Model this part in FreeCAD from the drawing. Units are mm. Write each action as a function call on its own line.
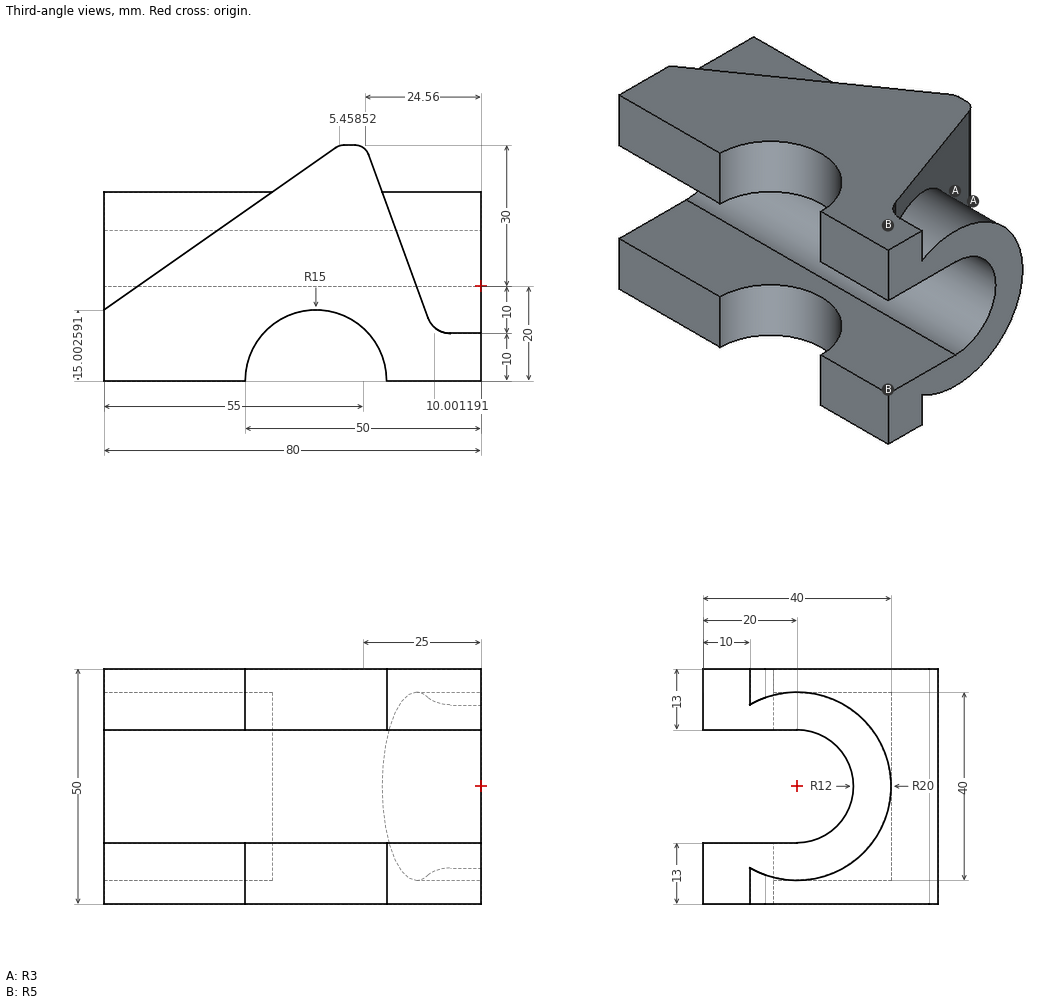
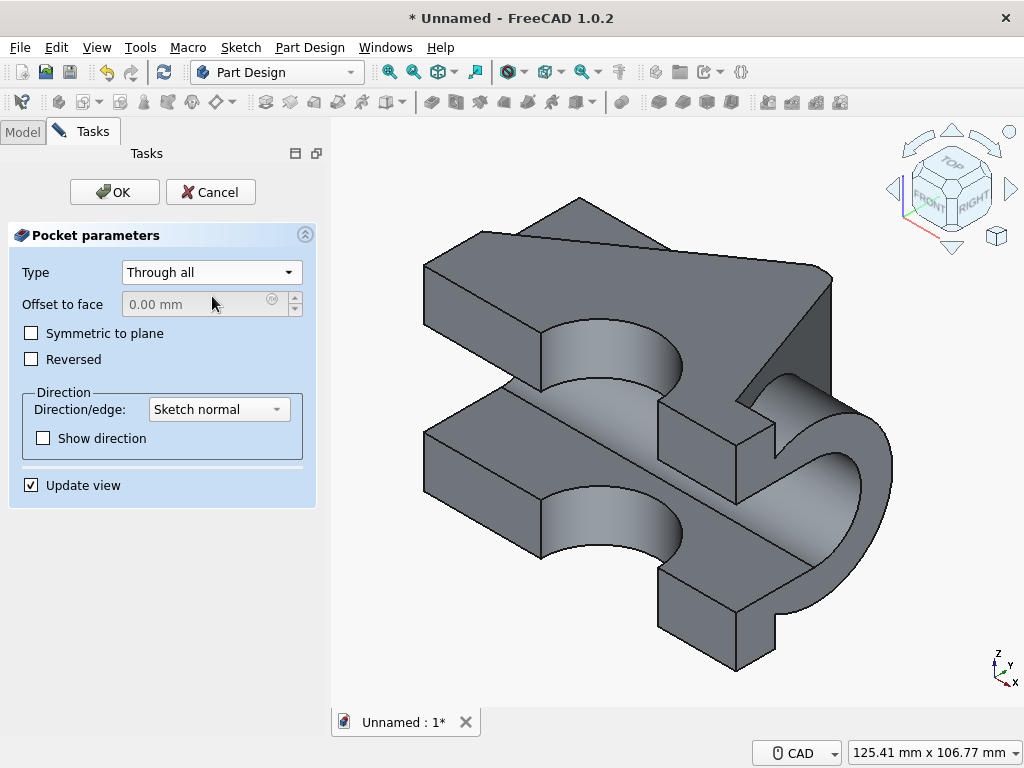
click(115, 192)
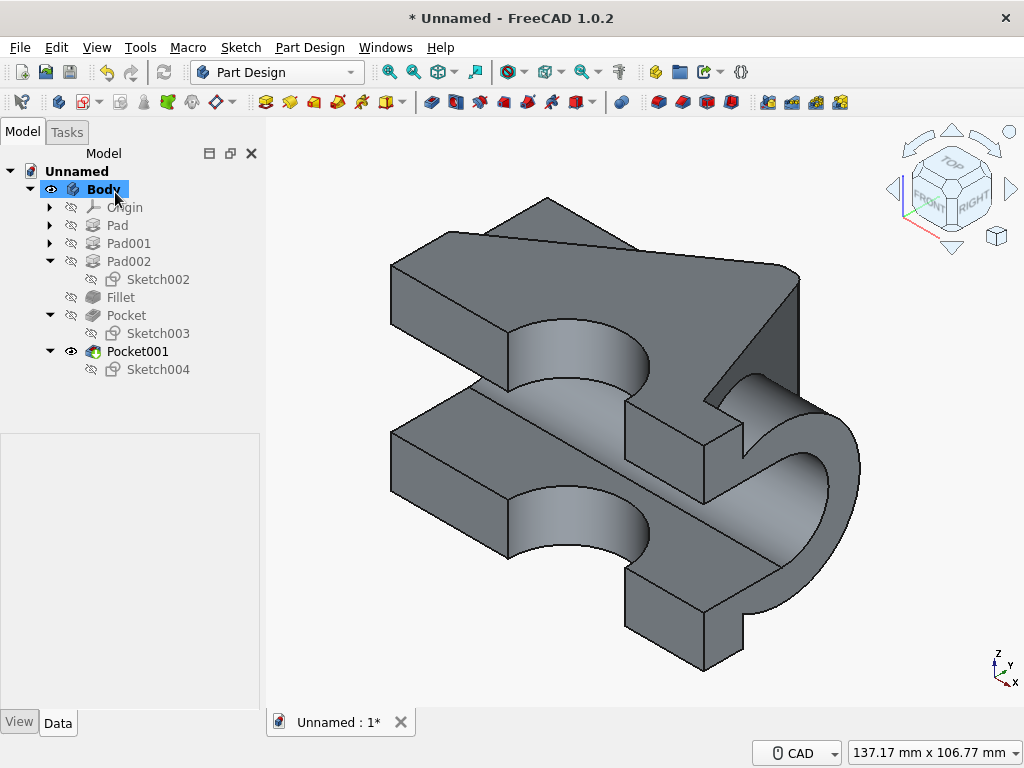
key(2)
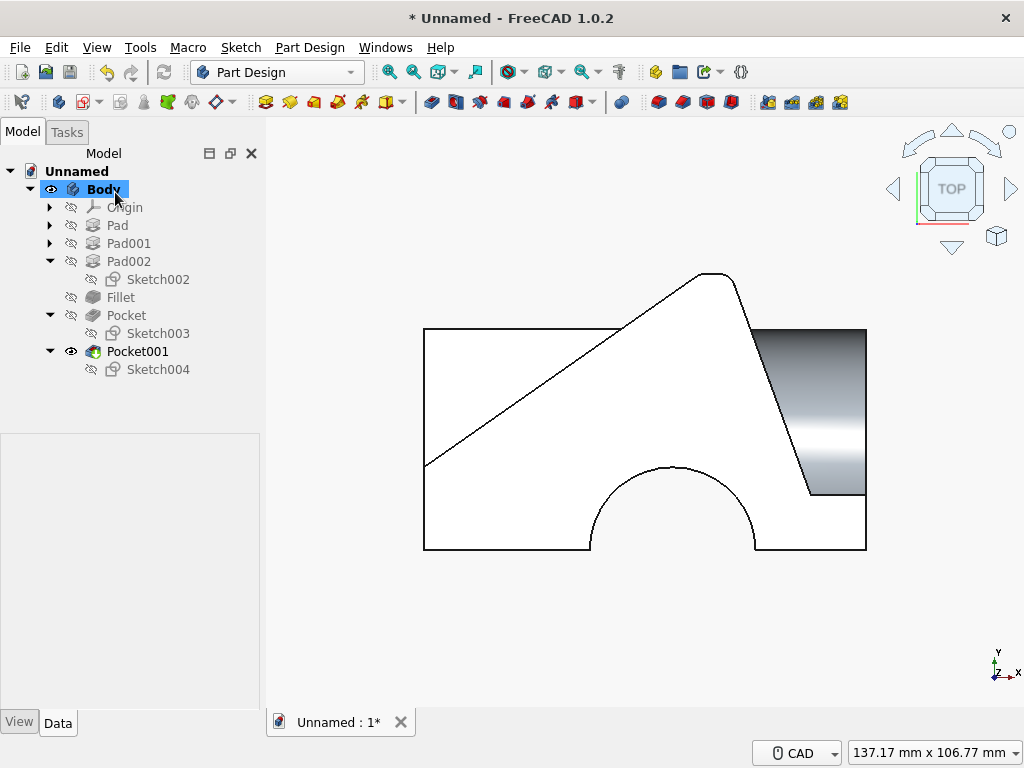
key(0)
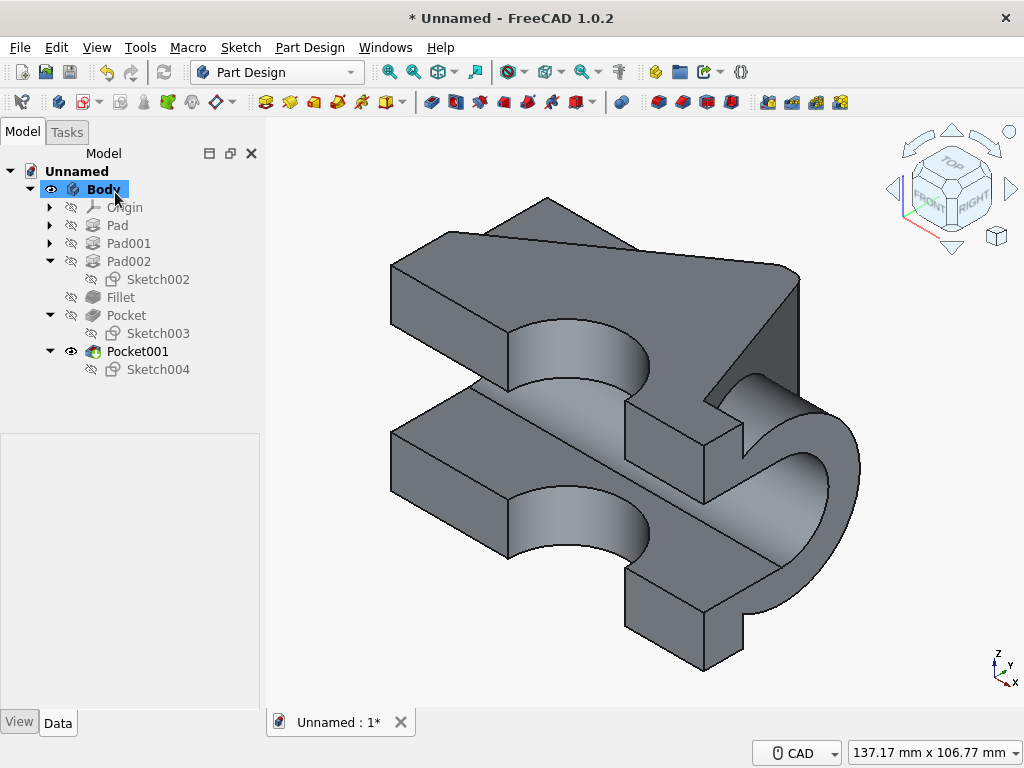
key(1)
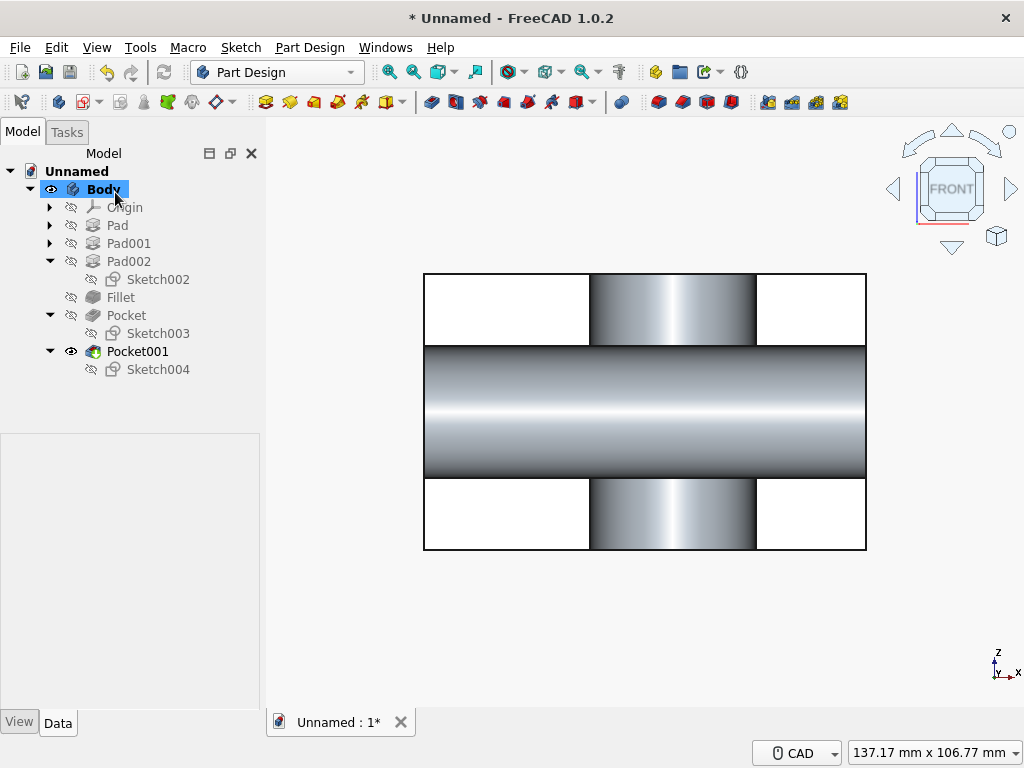
key(3)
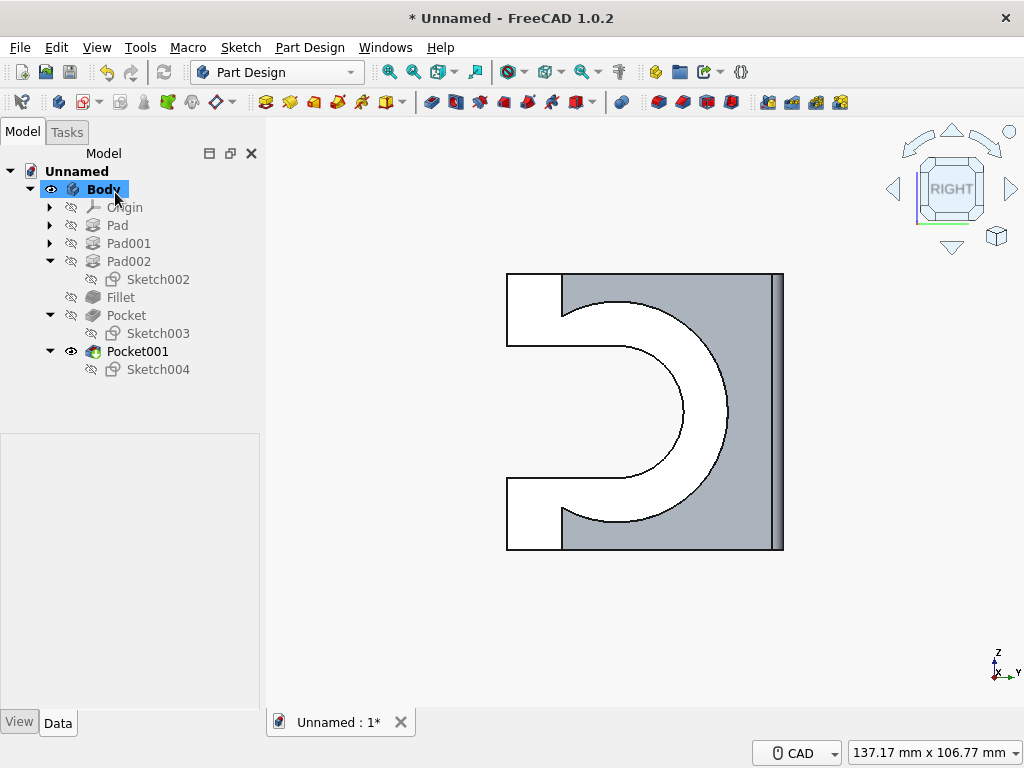
key(5)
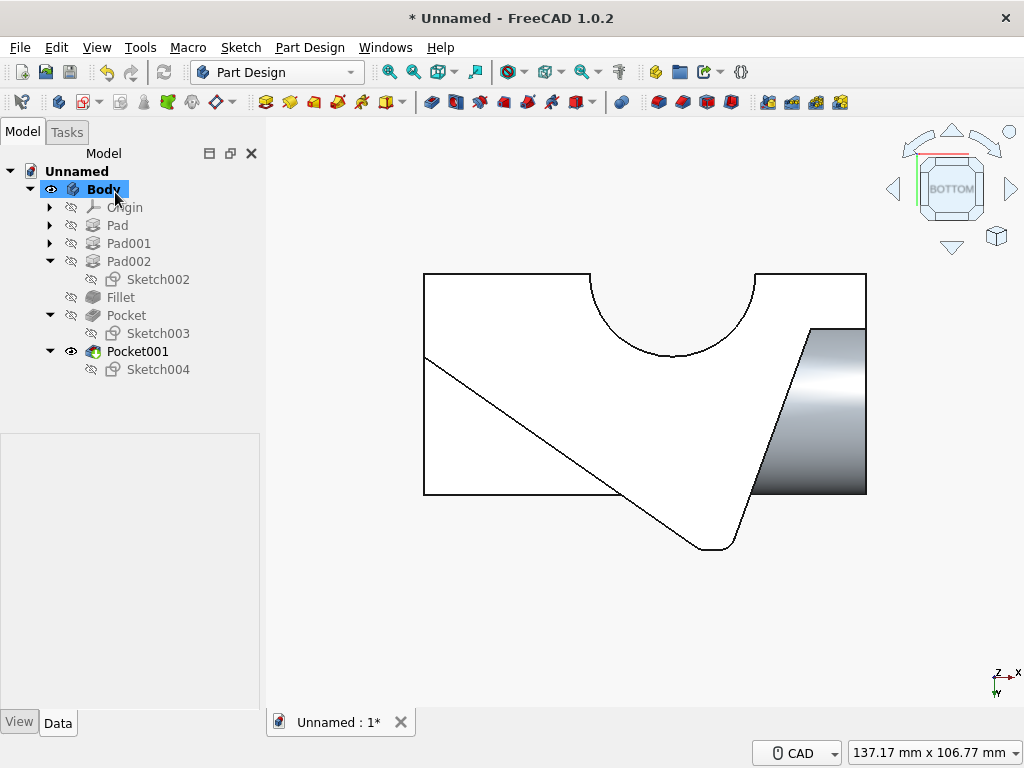
key(4)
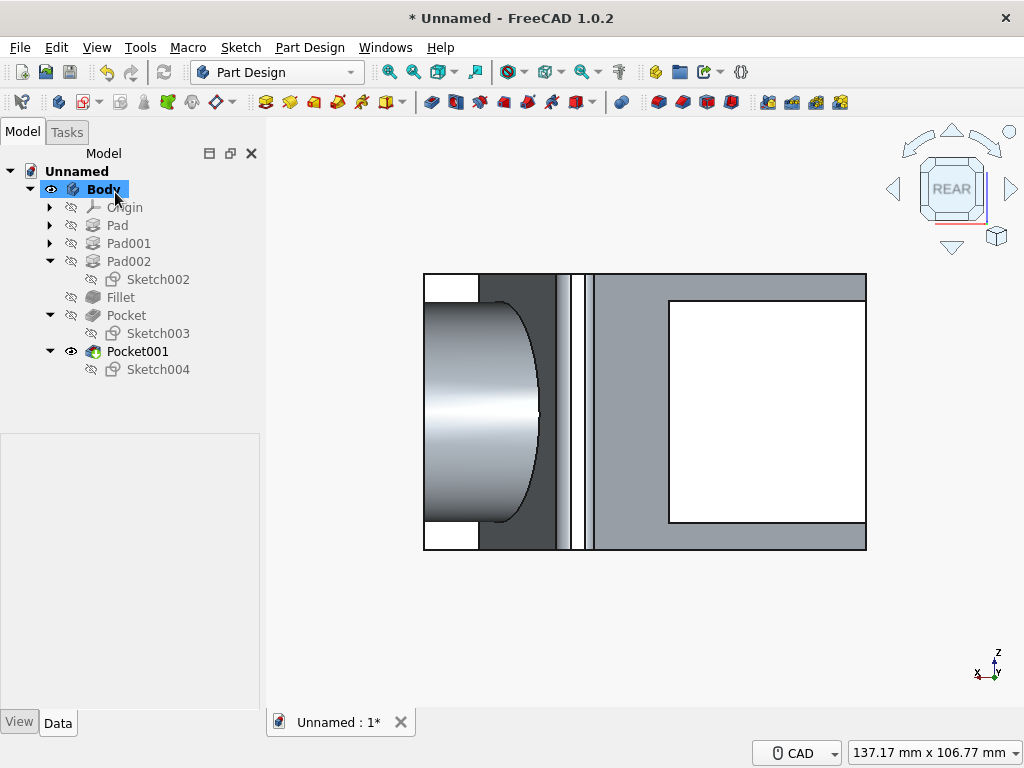
key(6)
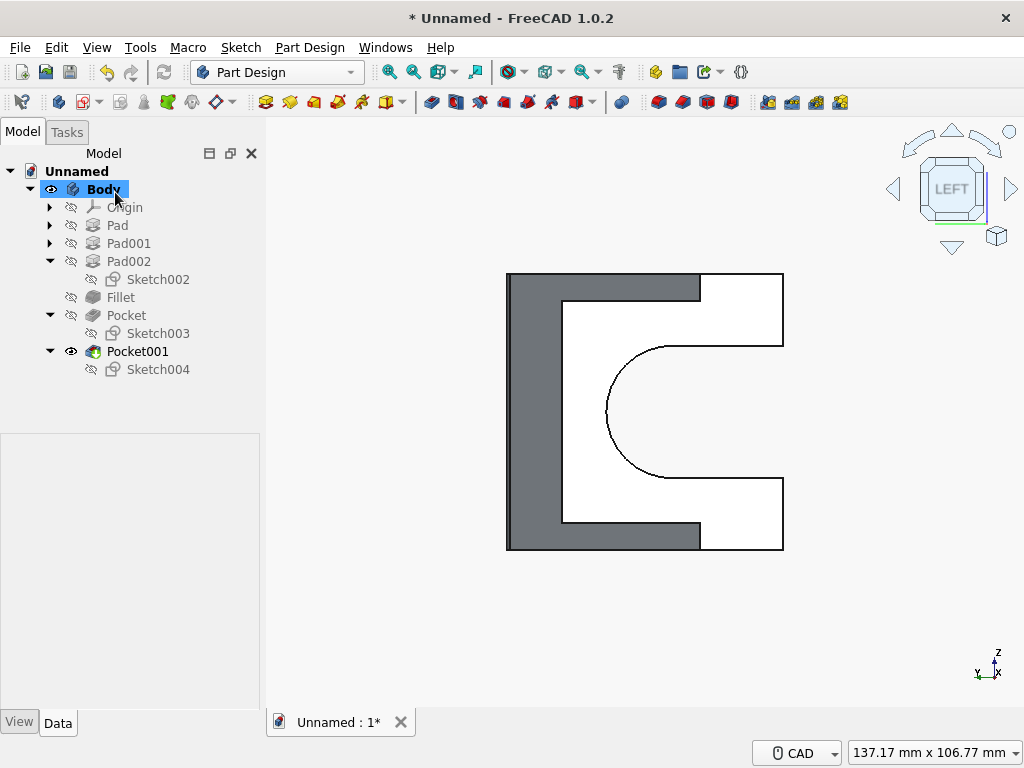
key(v)
key(3)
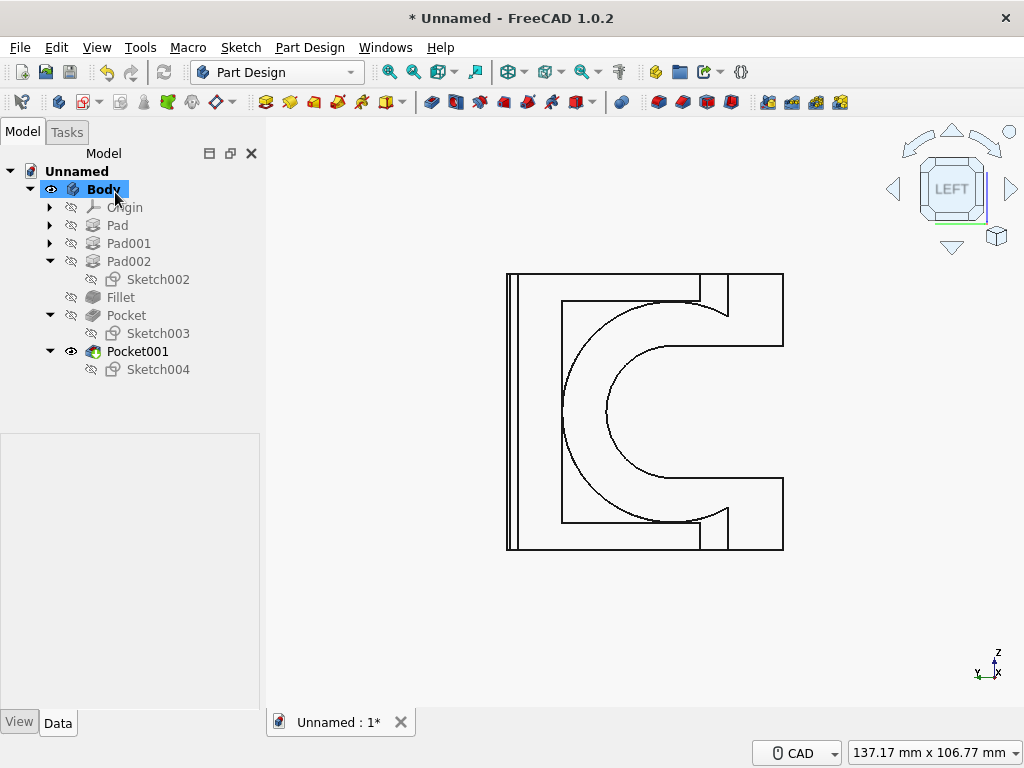
key(0)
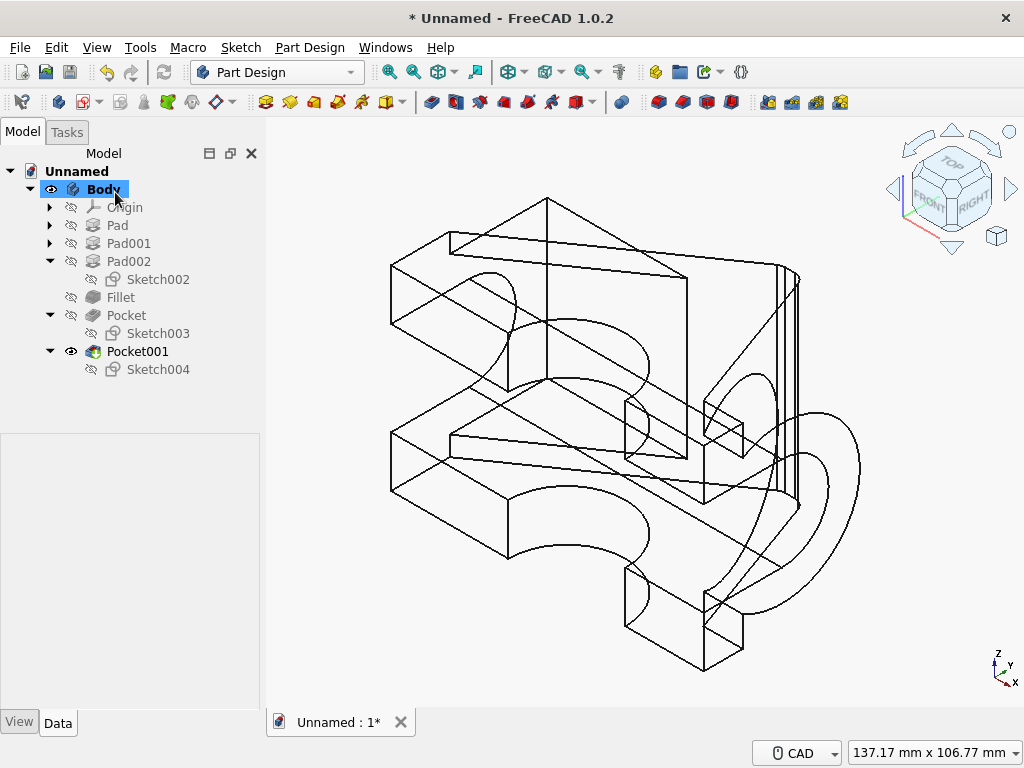
click(704, 601)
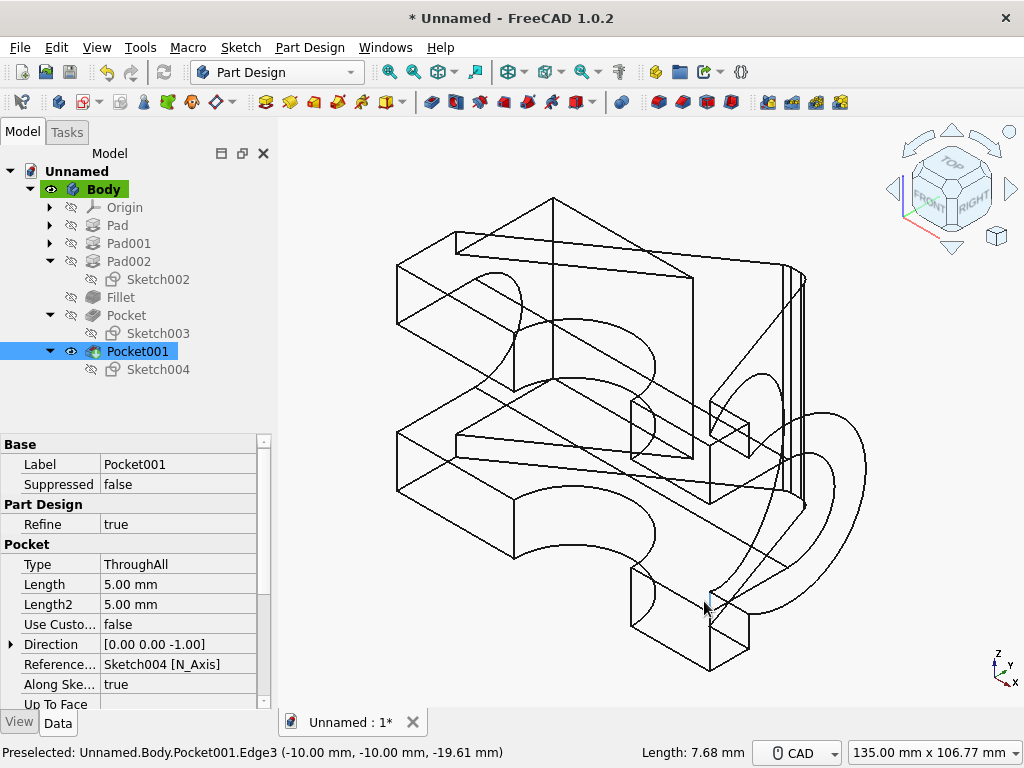
click(710, 417, ctrl)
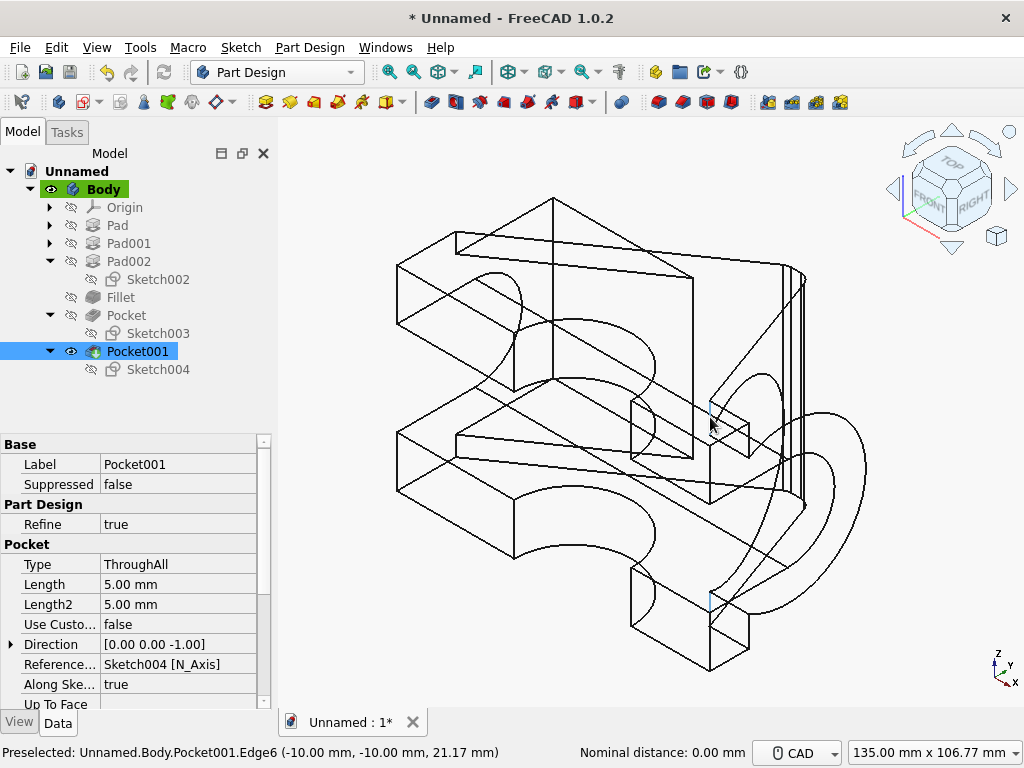
key(v)
key(1)